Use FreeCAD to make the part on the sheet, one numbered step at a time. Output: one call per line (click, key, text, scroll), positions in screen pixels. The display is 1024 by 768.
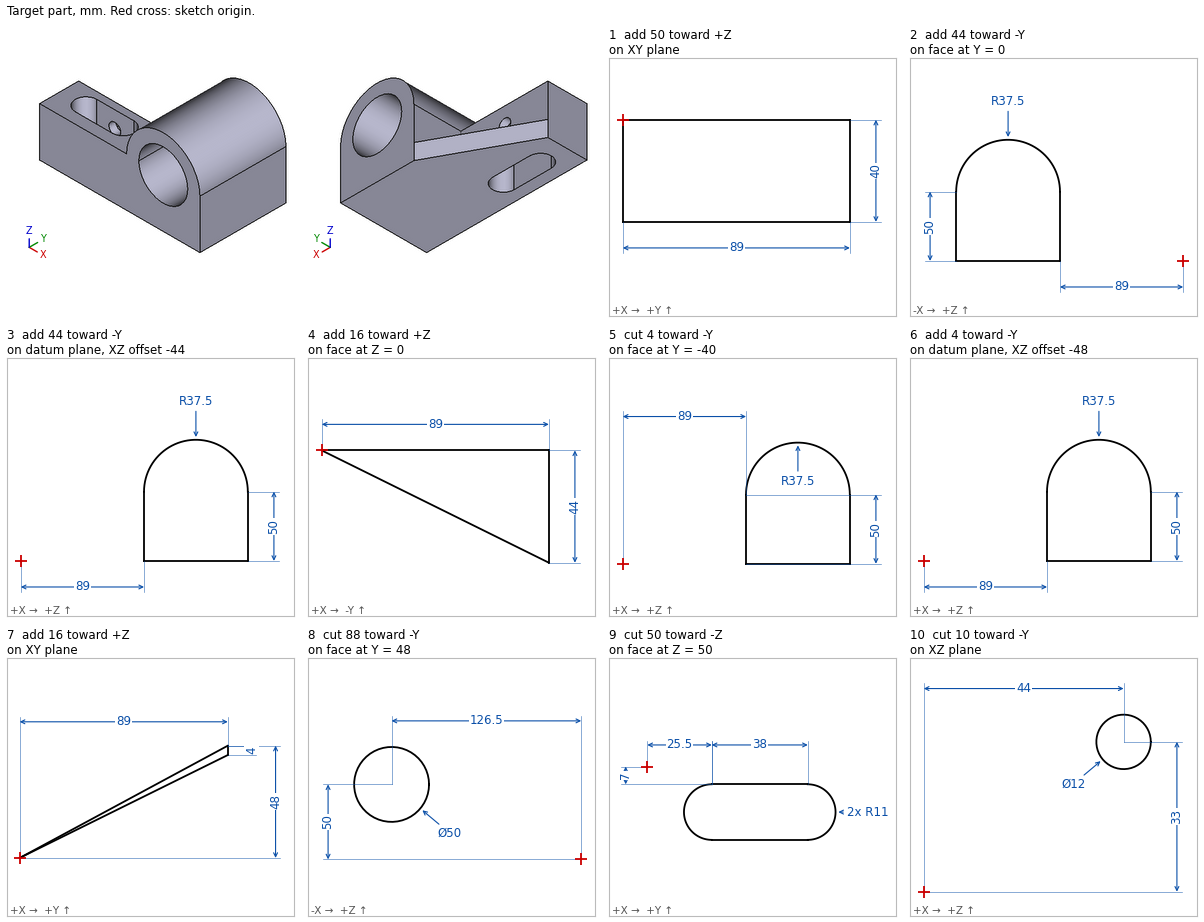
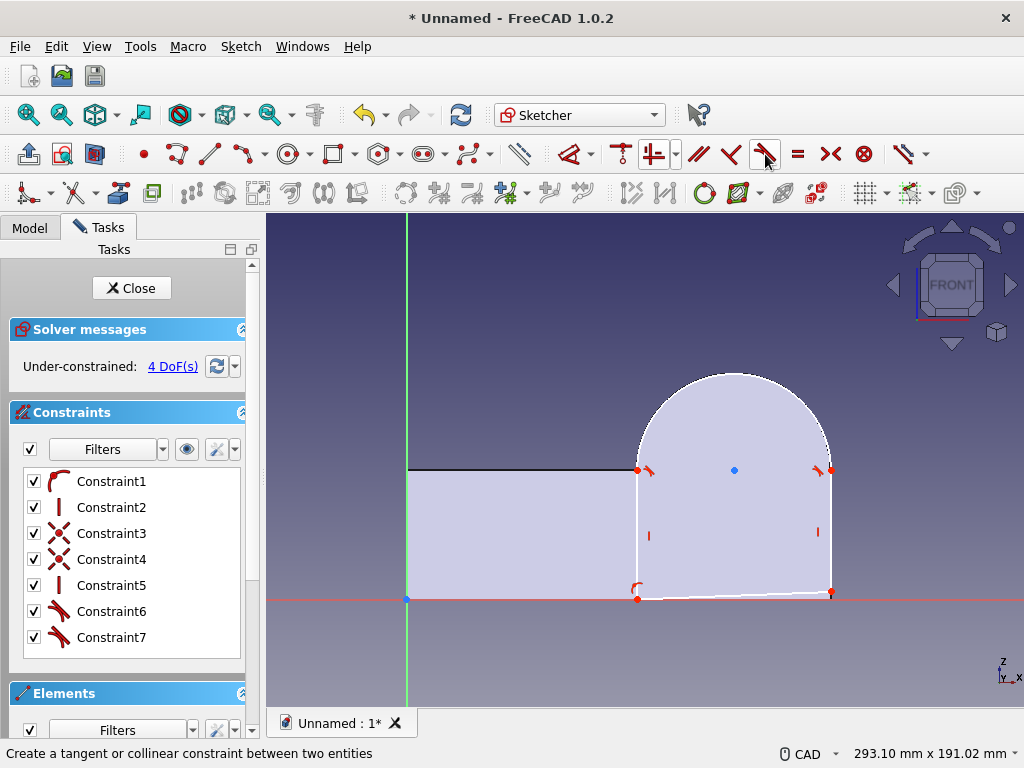
click(695, 597)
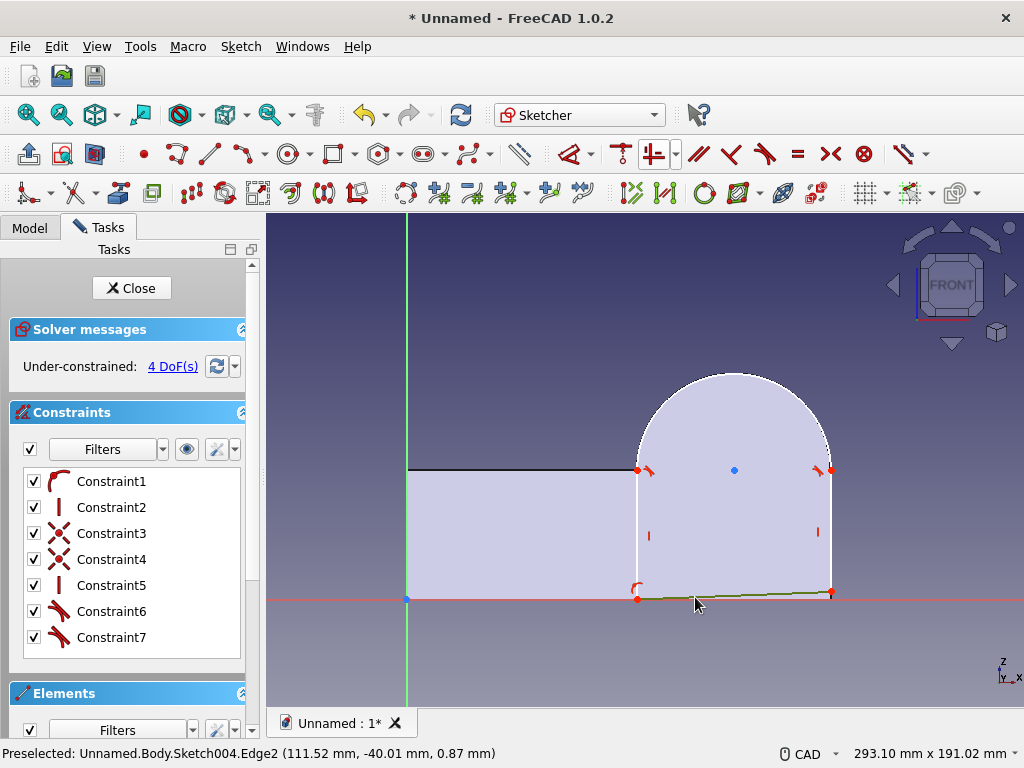
click(676, 154)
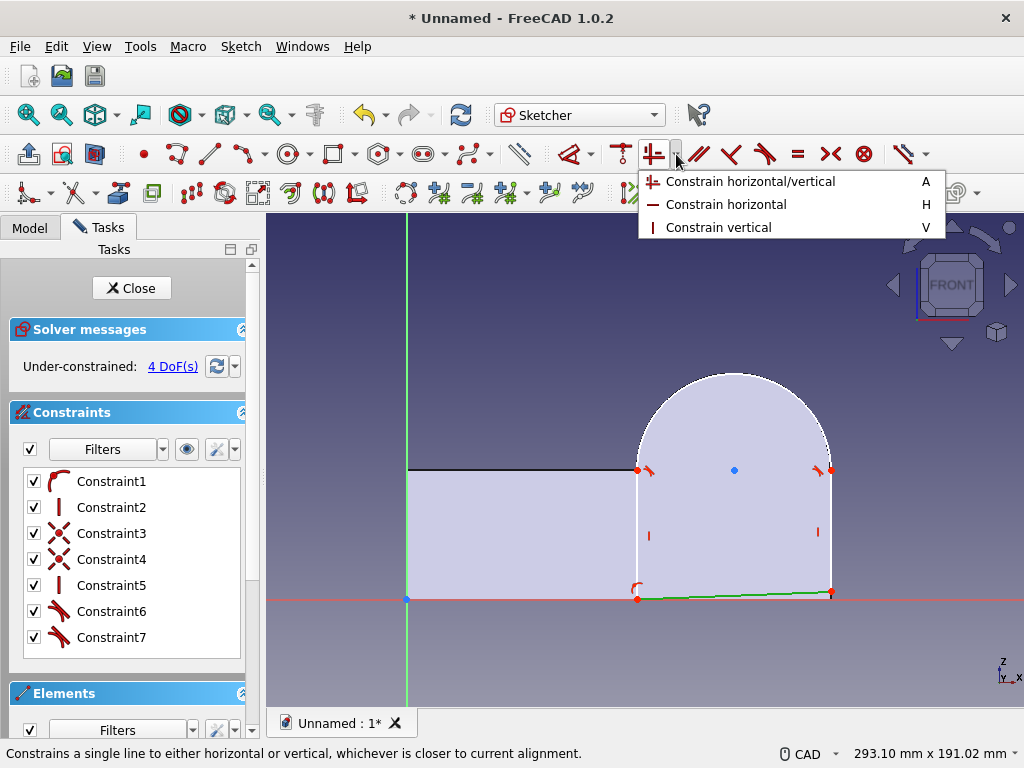
click(792, 204)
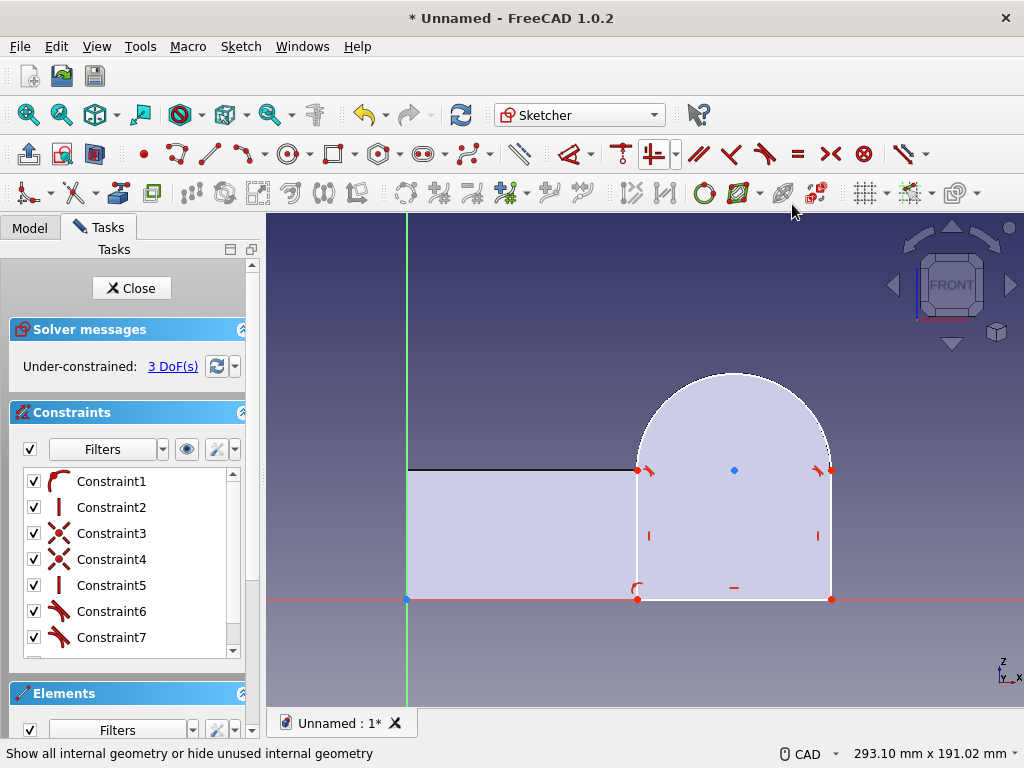
click(568, 154)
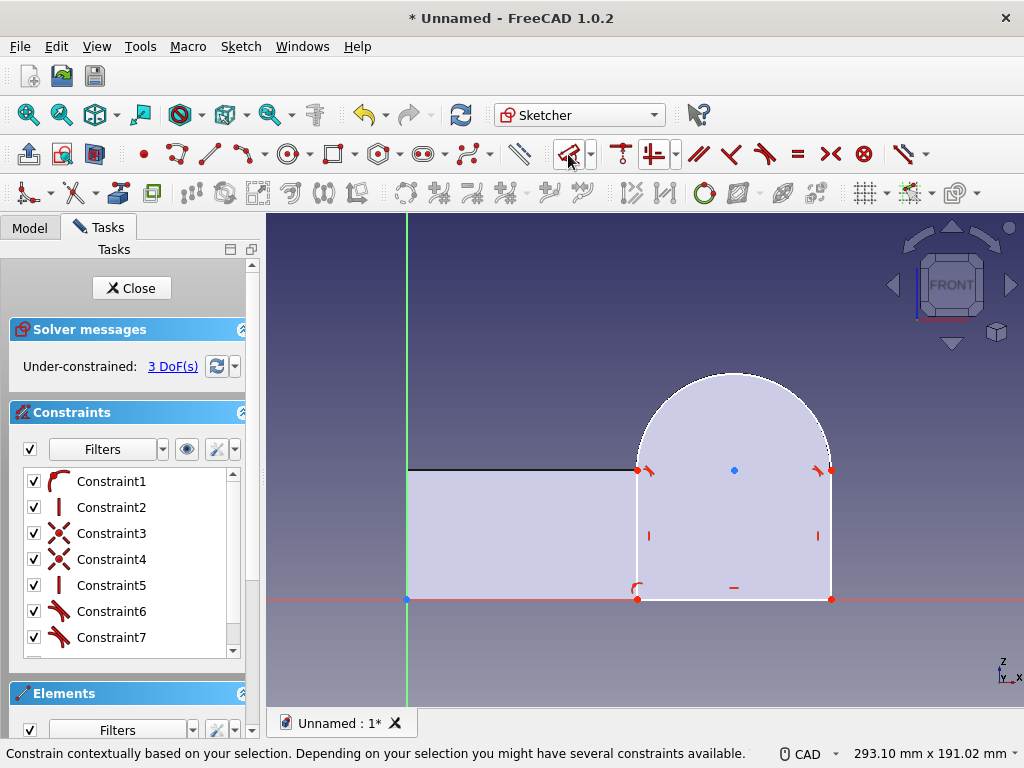
click(791, 393)
click(810, 367)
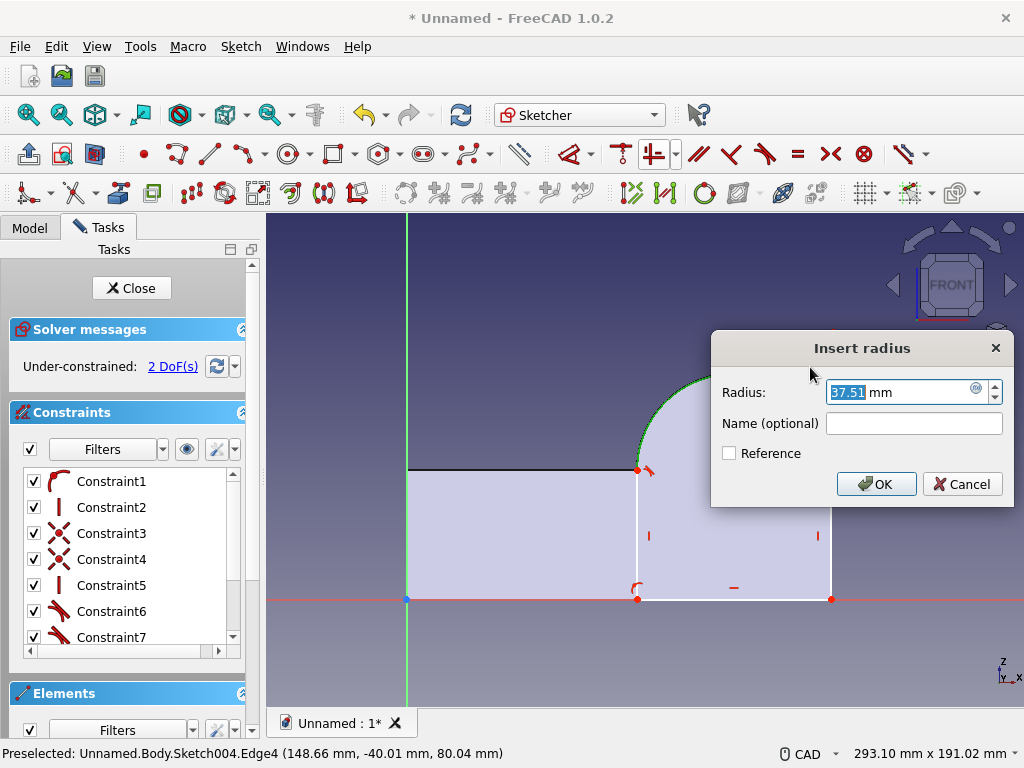
text(37.5)
key(Return)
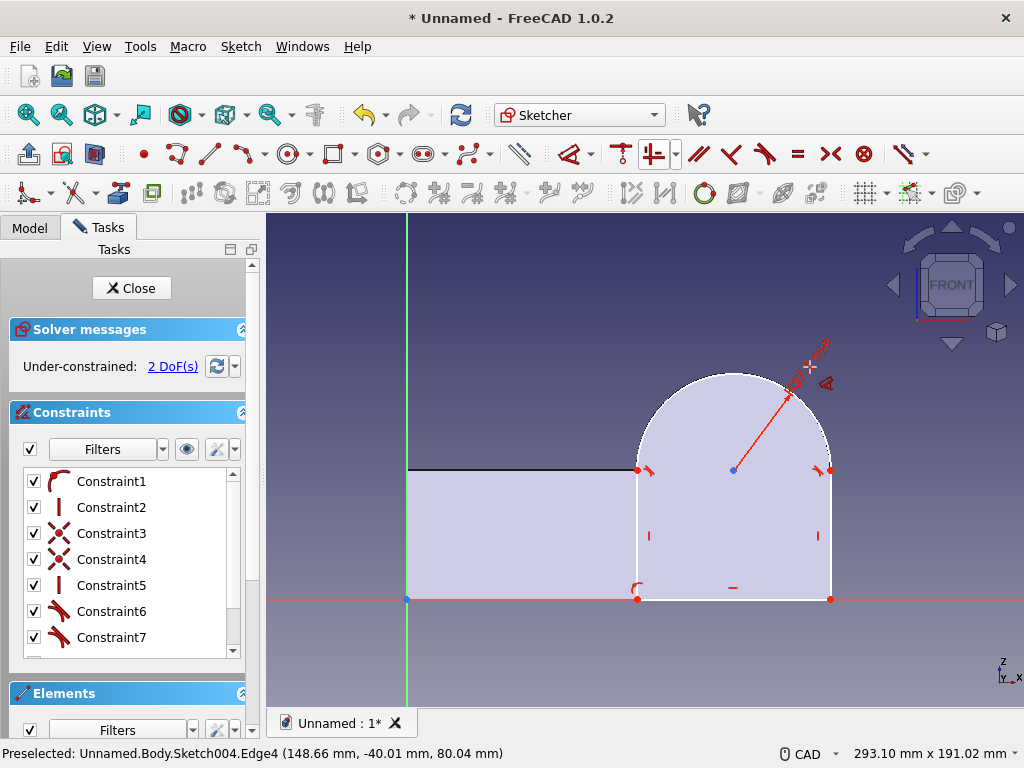
click(637, 510)
click(671, 535)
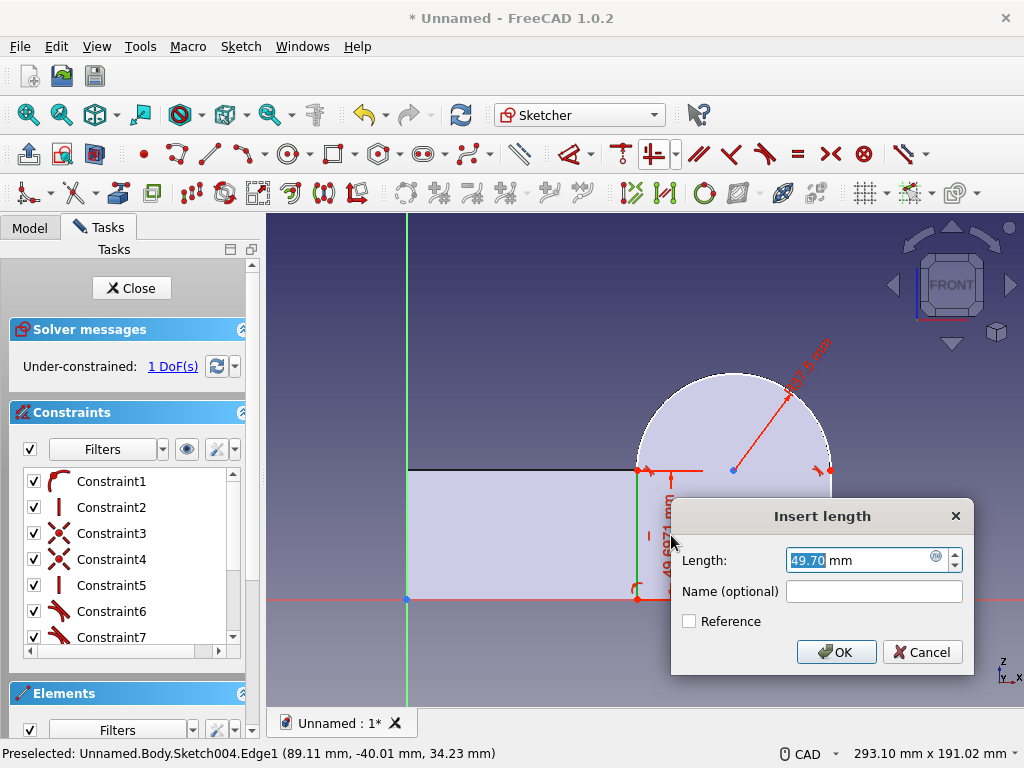
text(50)
key(Return)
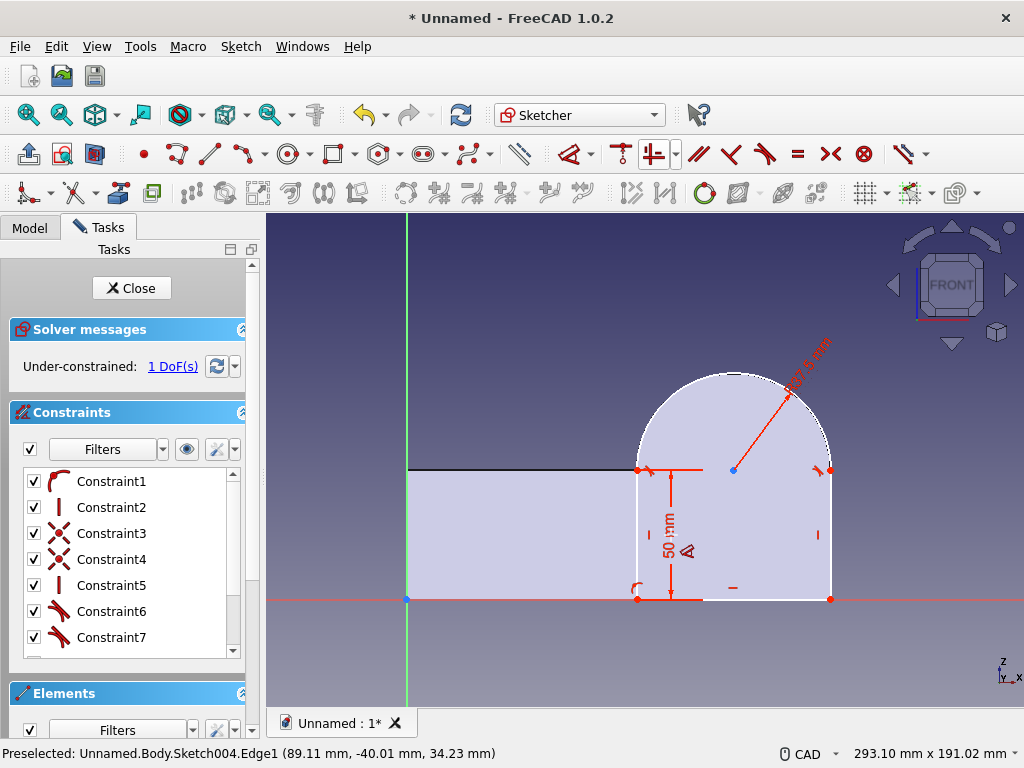
click(637, 470)
click(522, 634)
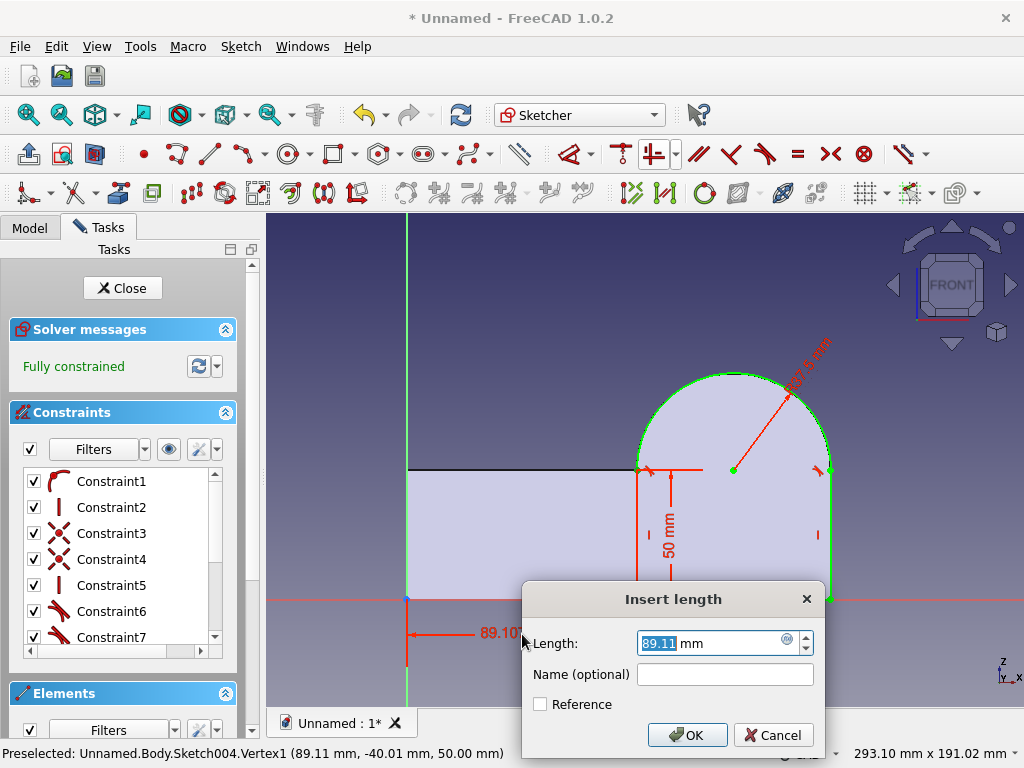
text(89)
key(Return)
key(Escape)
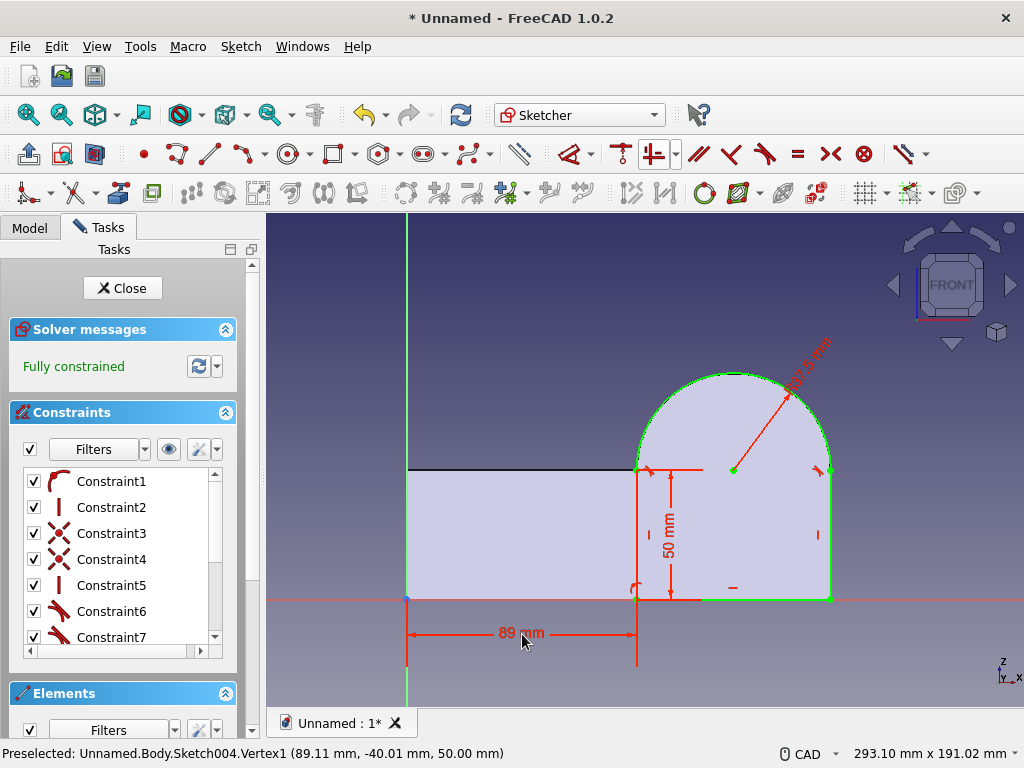
click(123, 288)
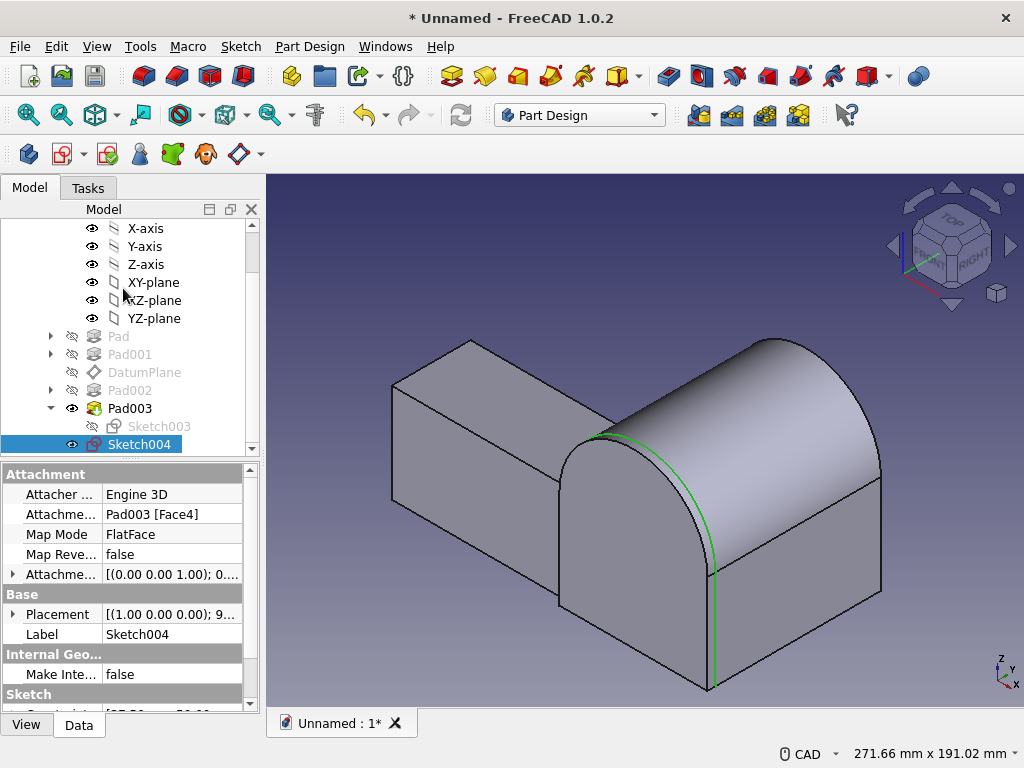
click(669, 76)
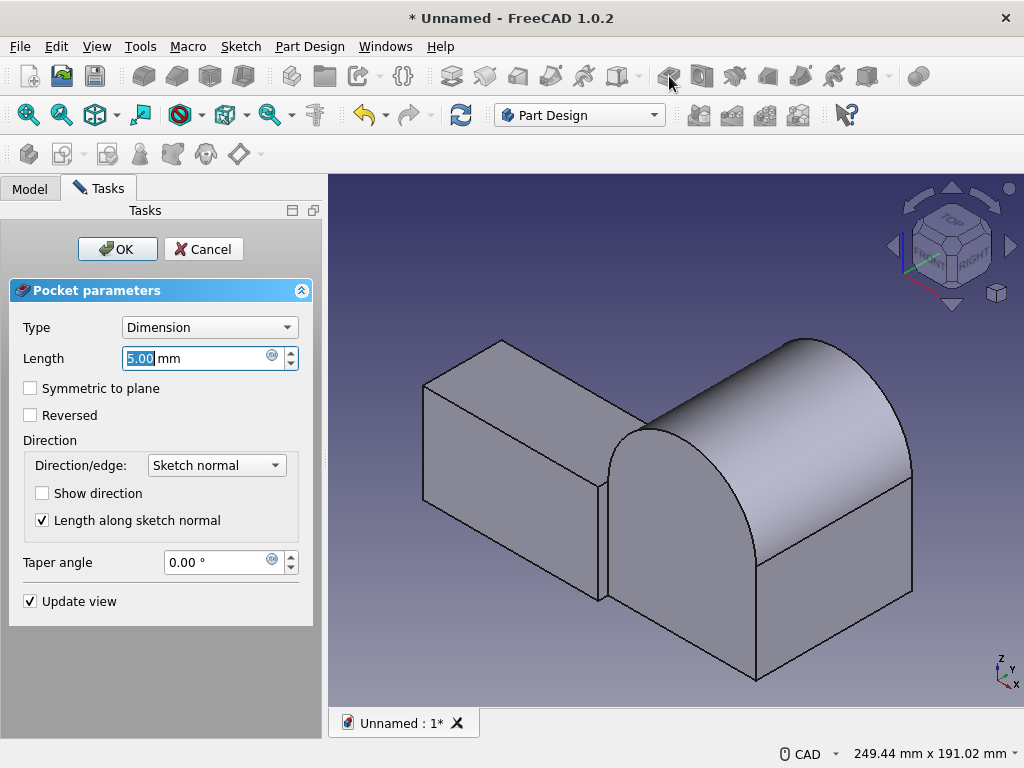
text(4)
key(Tab)